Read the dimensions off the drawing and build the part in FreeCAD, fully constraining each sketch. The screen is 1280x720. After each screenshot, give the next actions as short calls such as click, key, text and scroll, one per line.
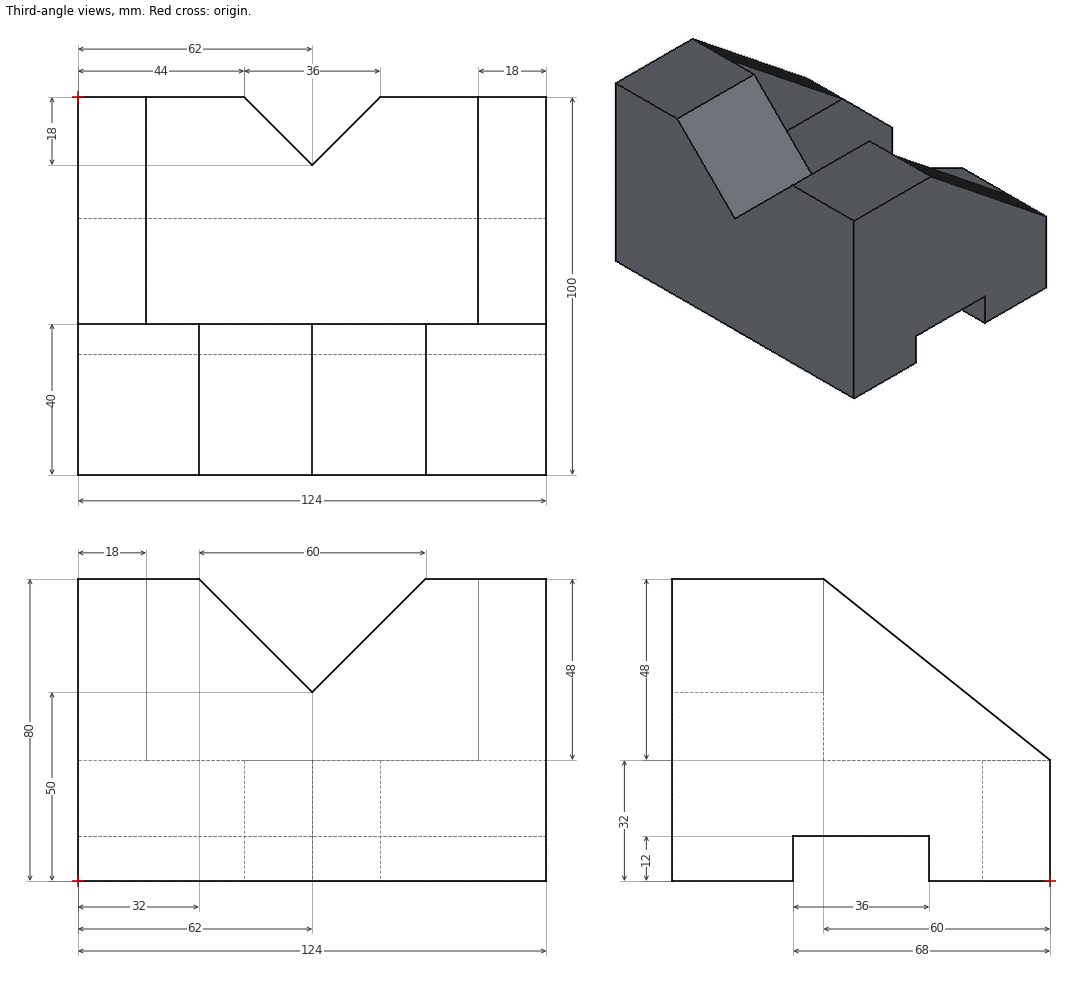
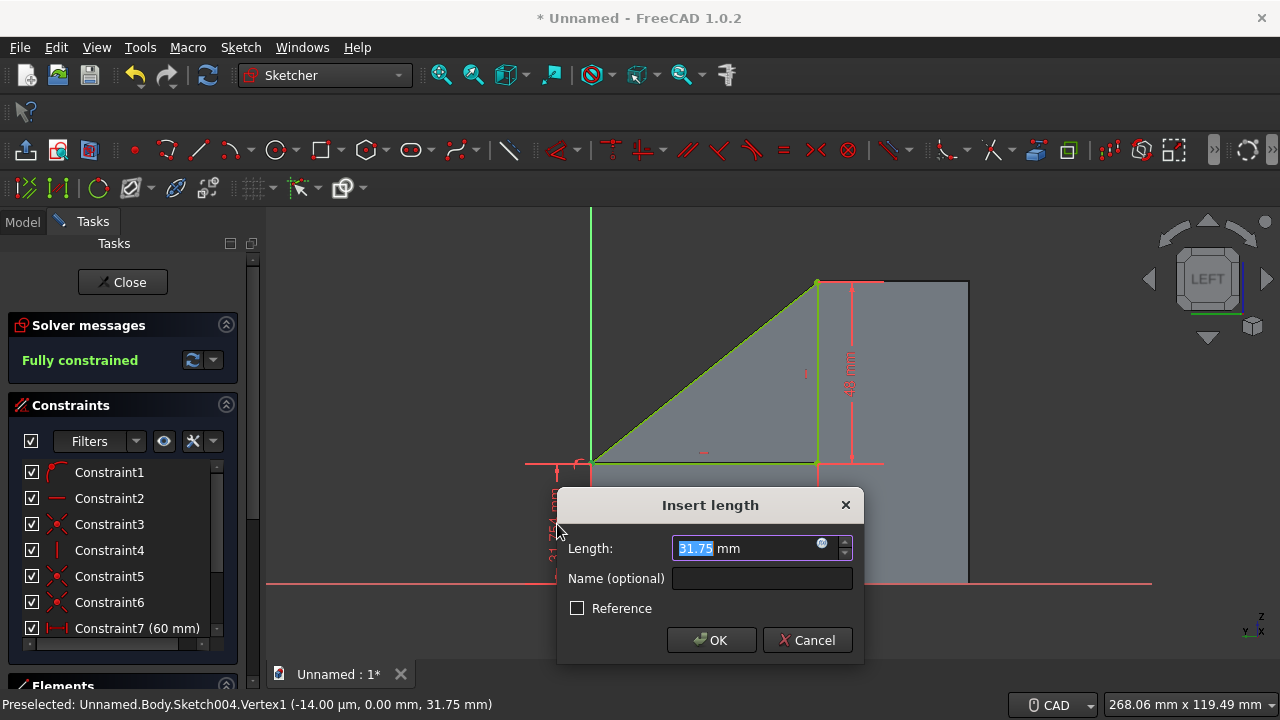
text(32)
key(Return)
key(Escape)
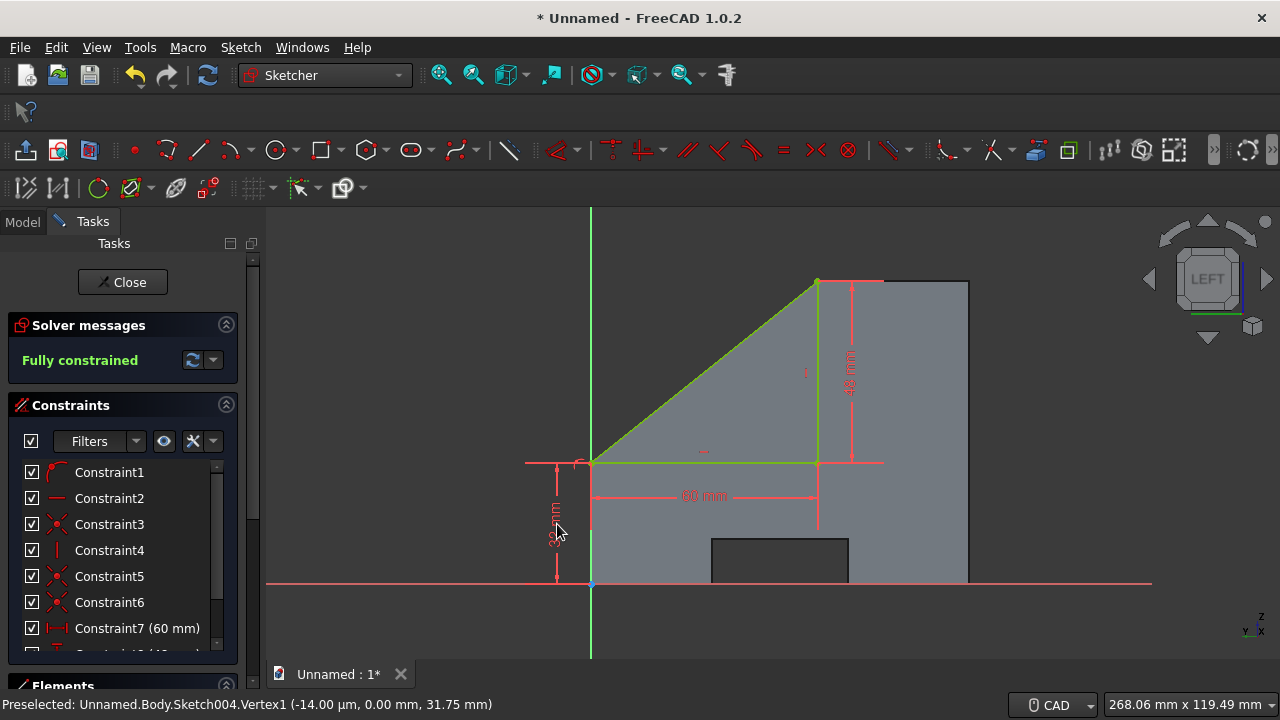
click(123, 282)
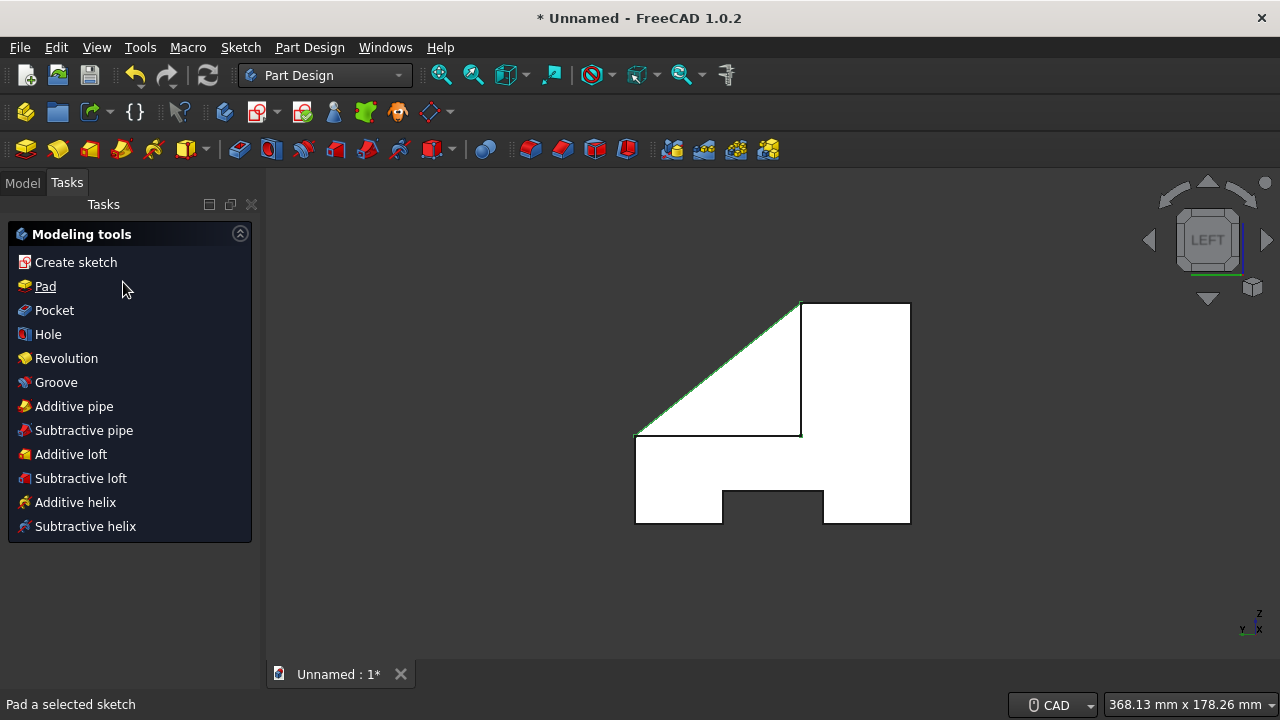
click(26, 150)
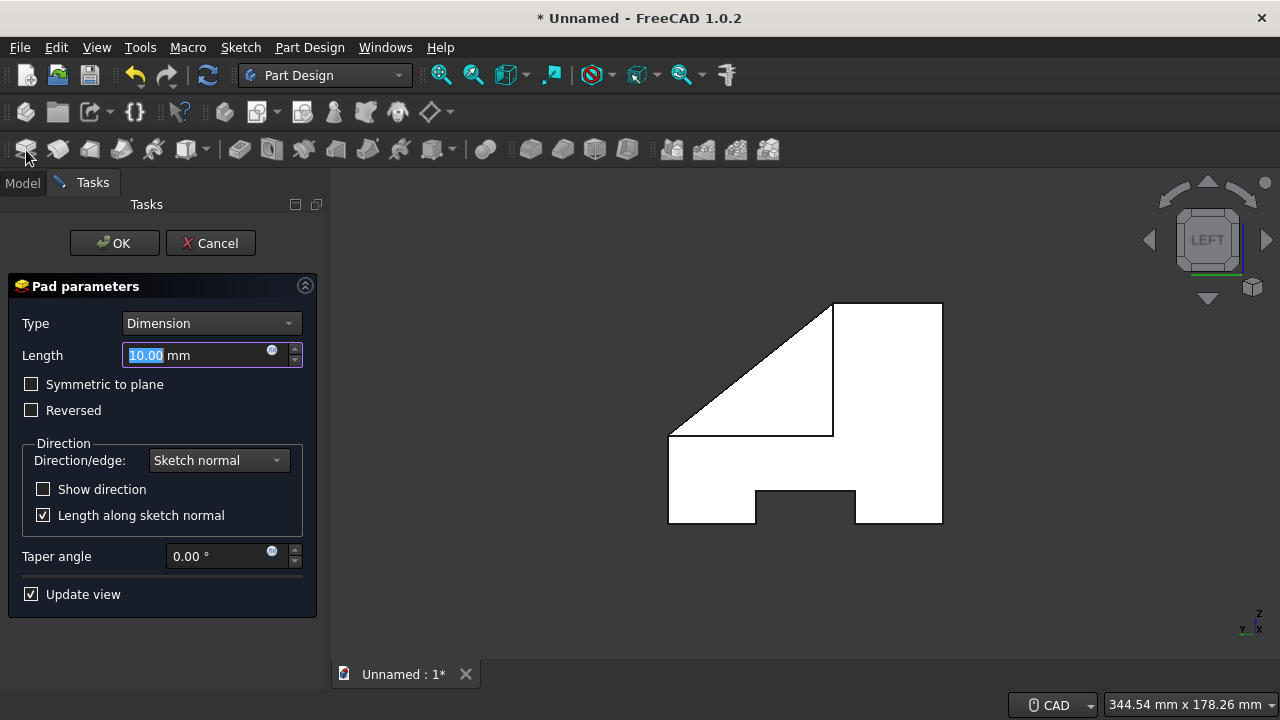
text(18)
key(Tab)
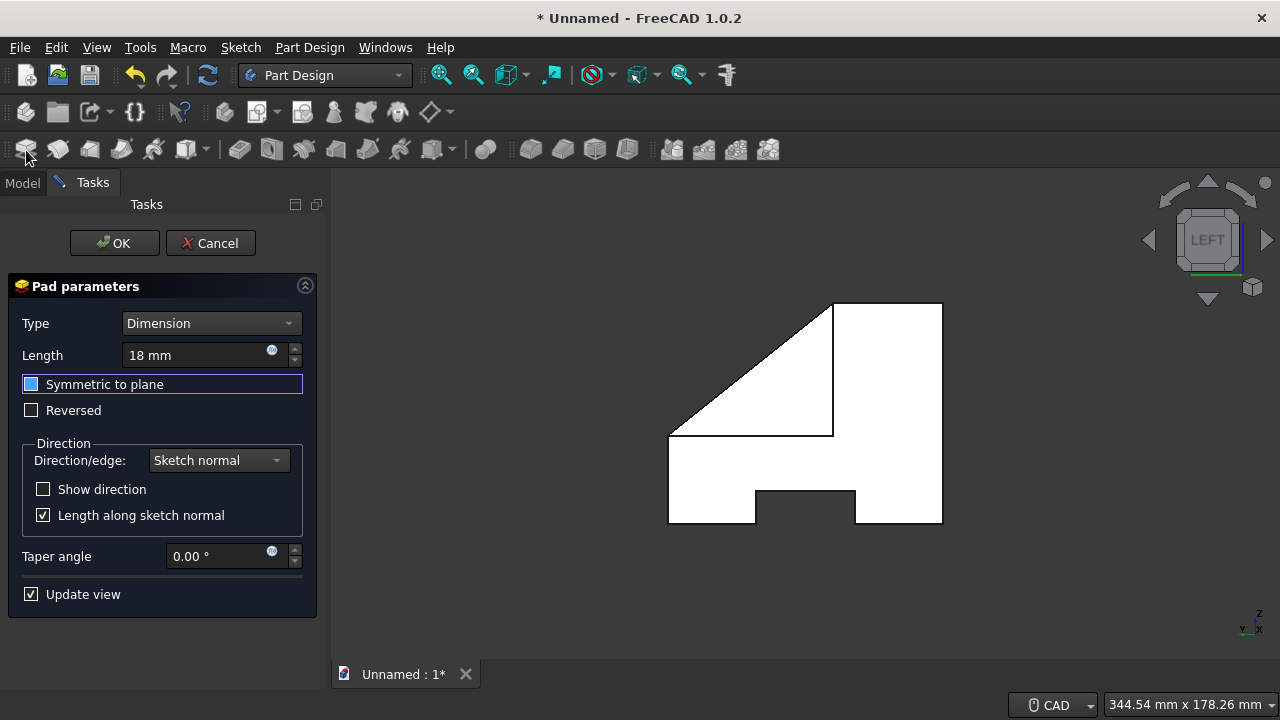
click(30, 410)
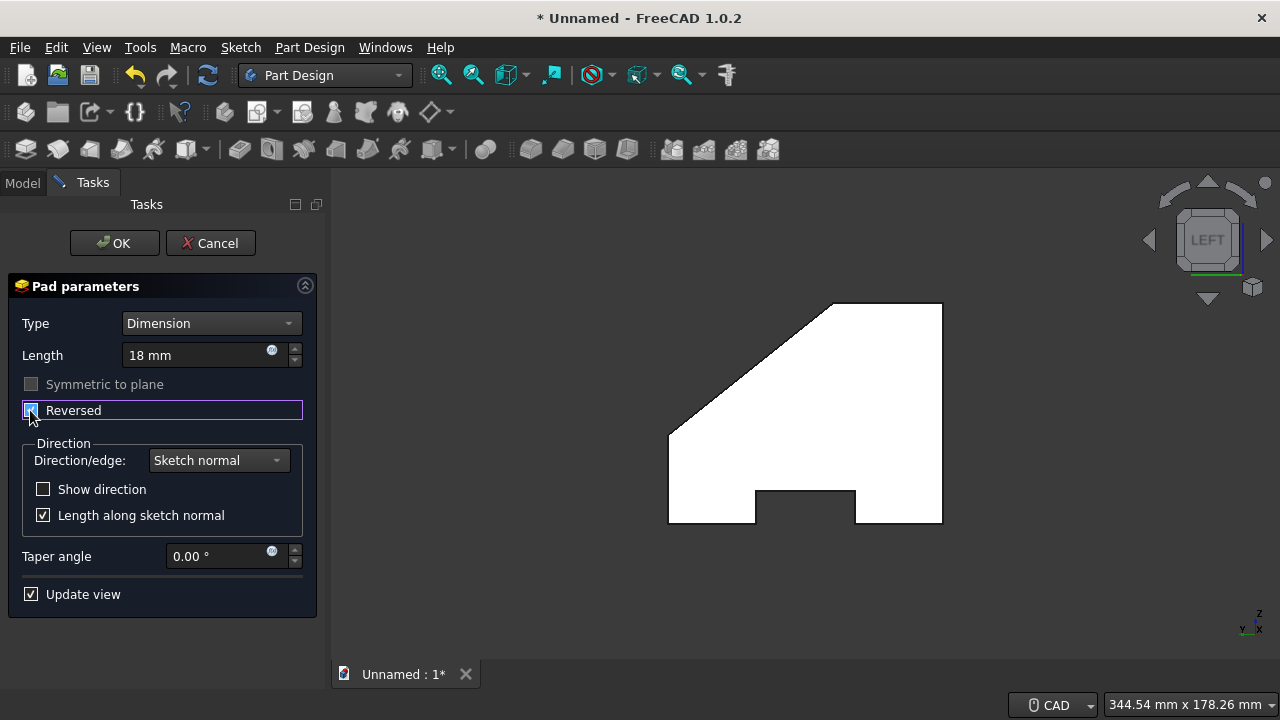
click(115, 243)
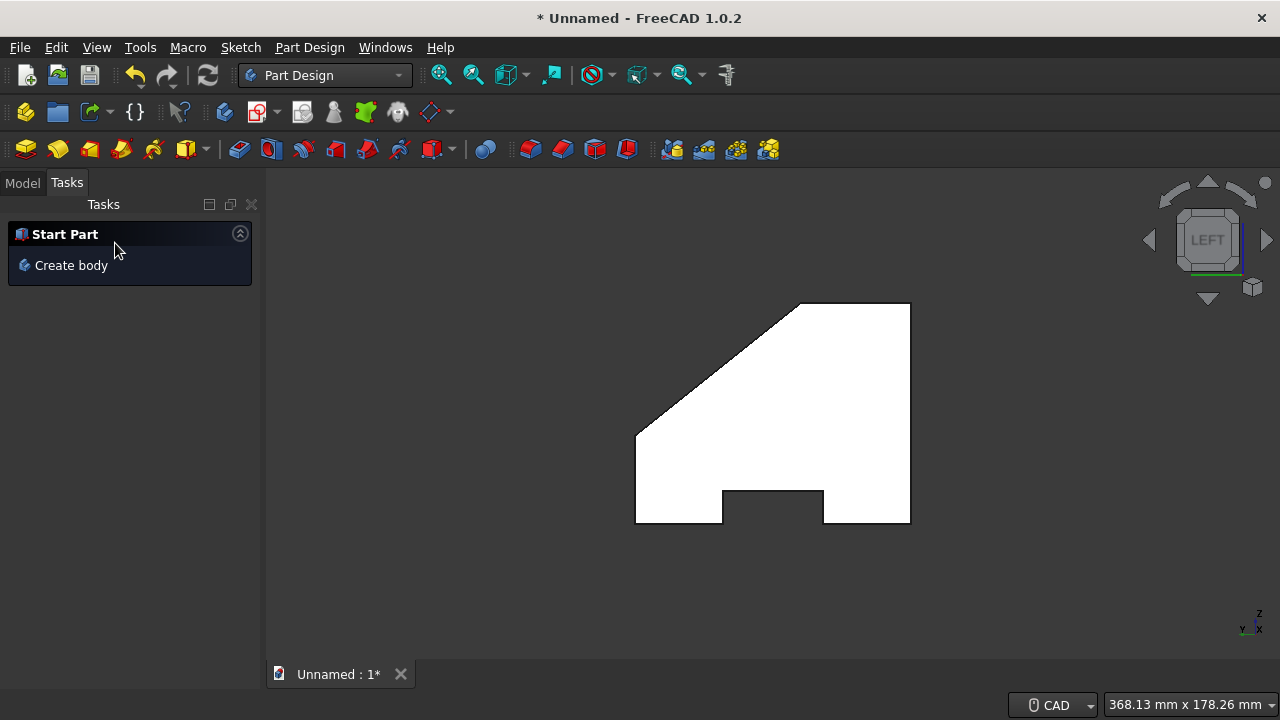
key(4)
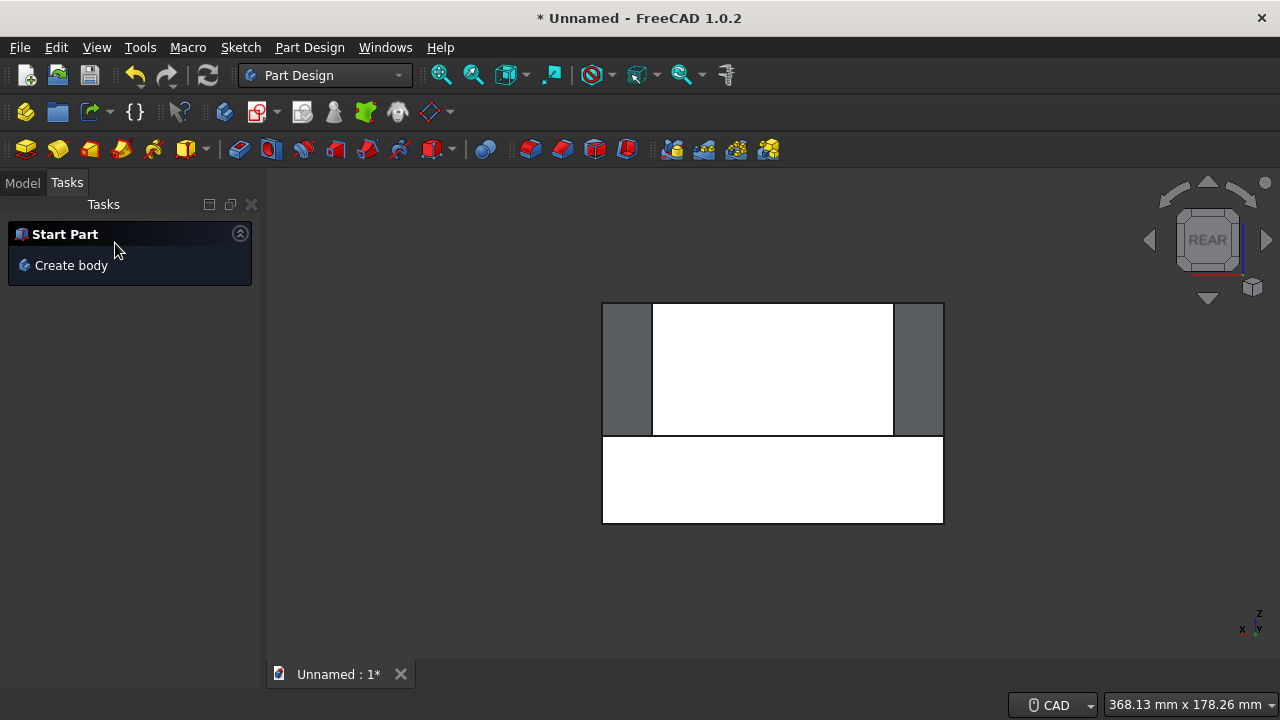
click(738, 368)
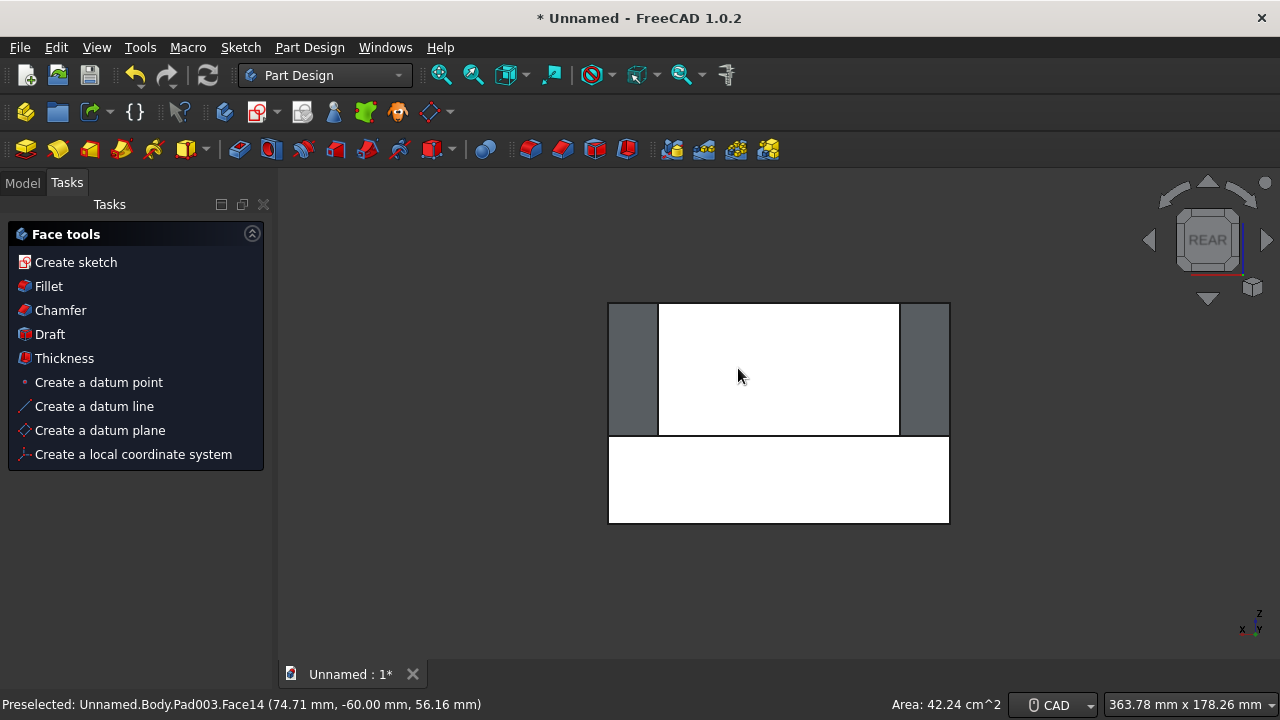
click(258, 112)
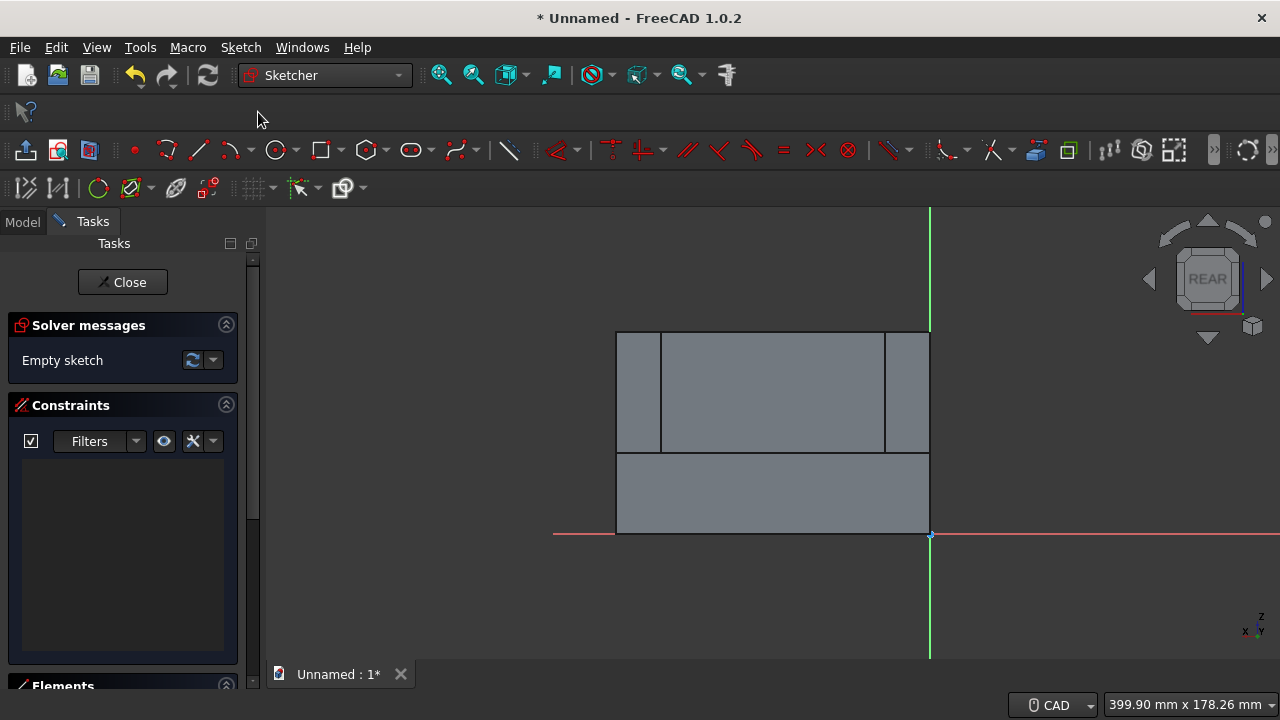
scroll(1035, 433, up, 2)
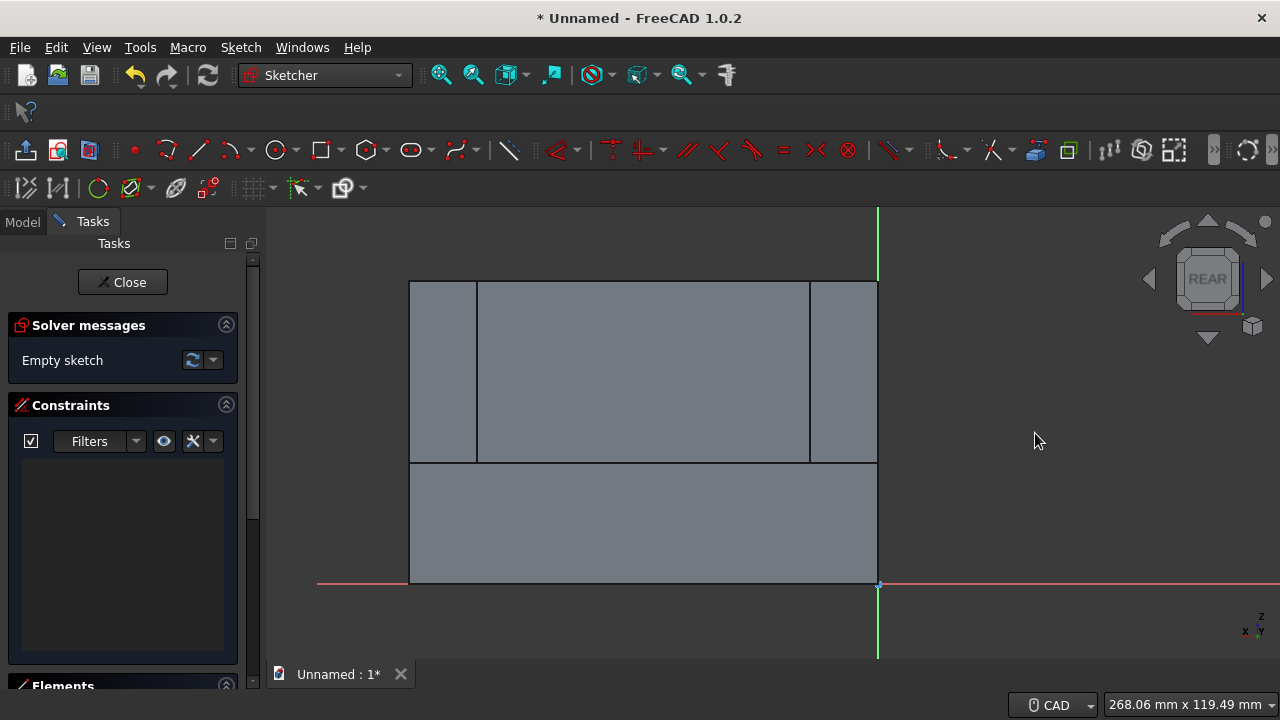
click(168, 150)